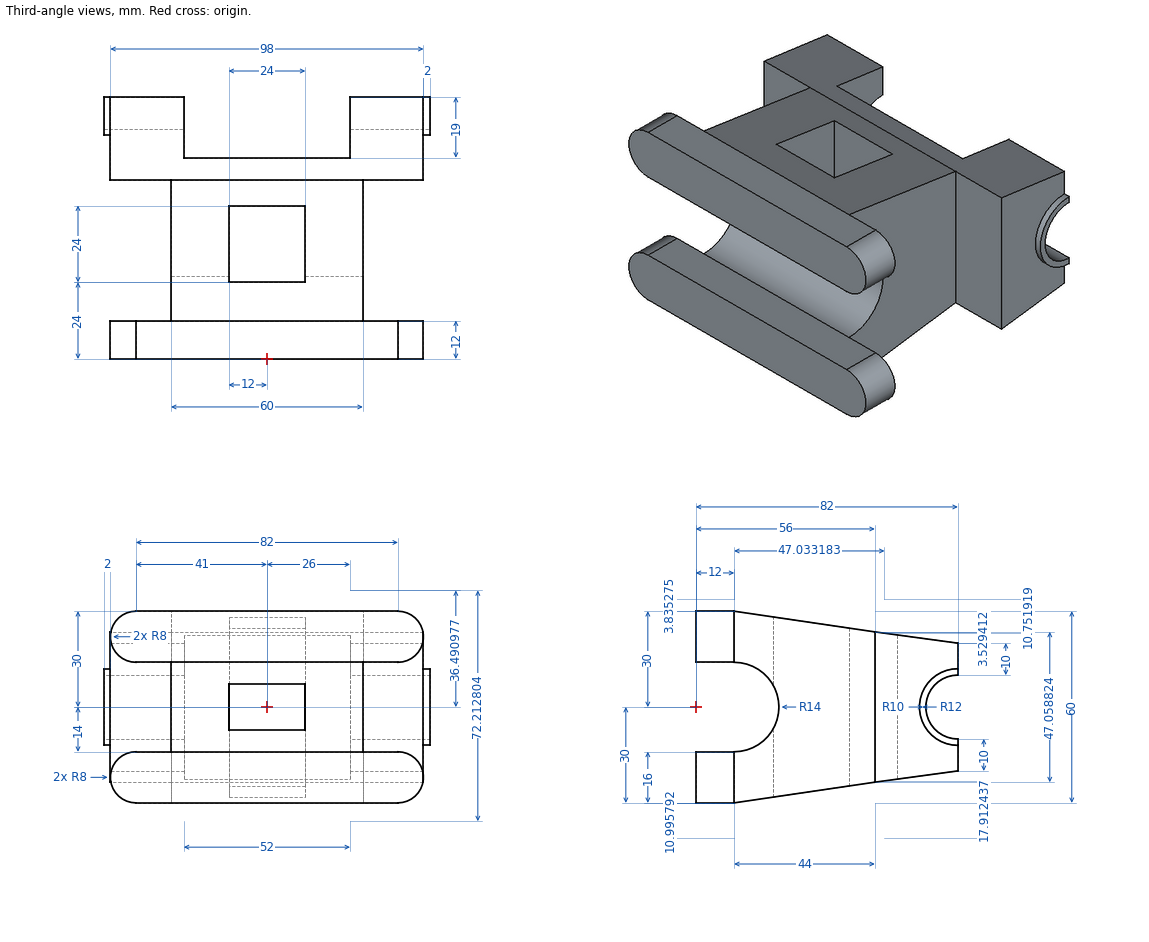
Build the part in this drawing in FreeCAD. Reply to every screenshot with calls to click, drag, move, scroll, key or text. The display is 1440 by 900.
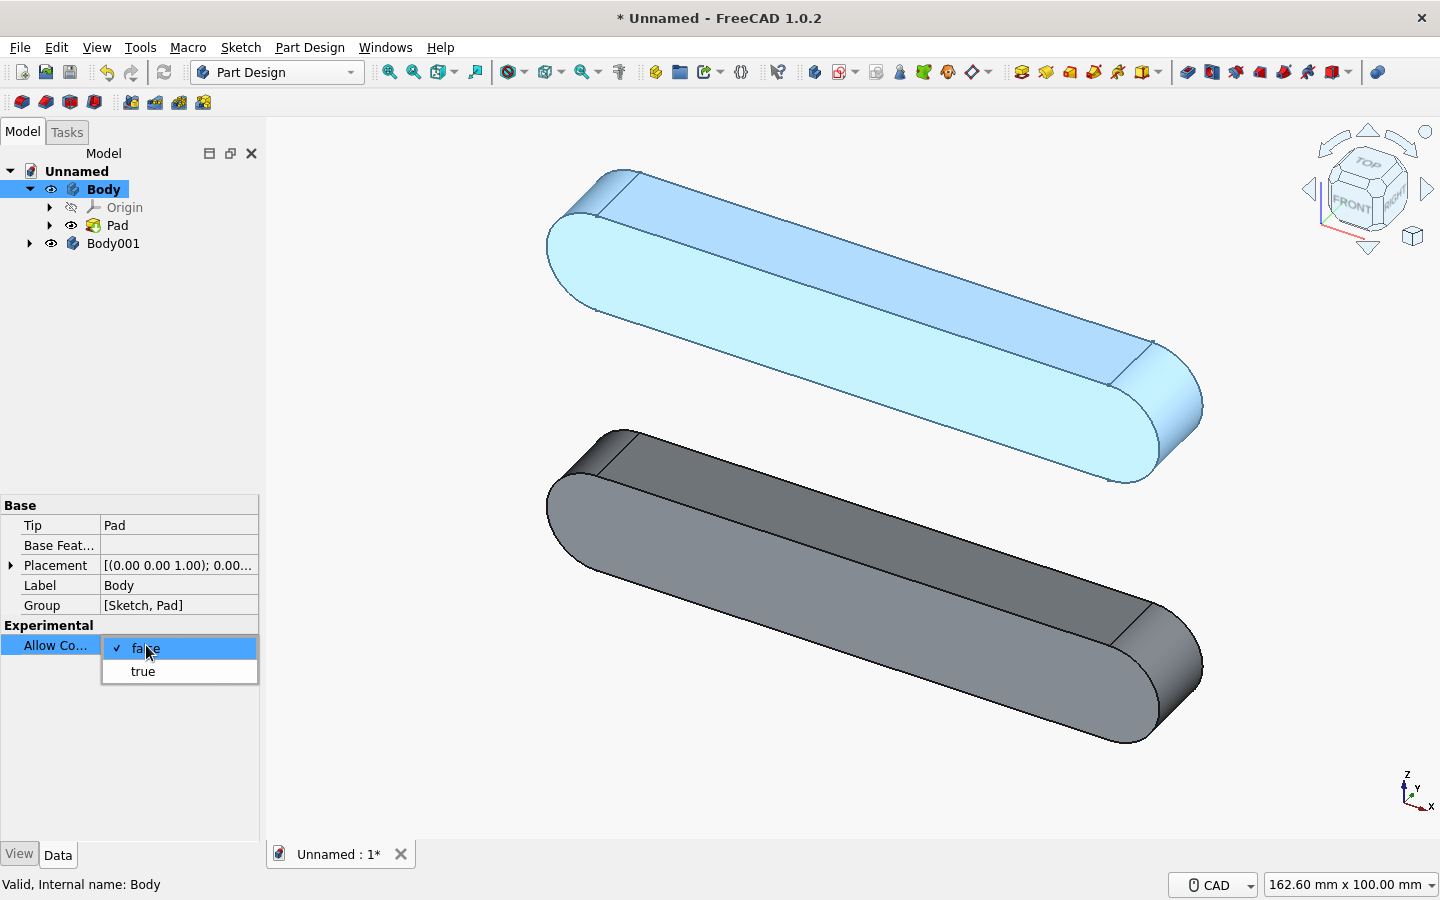
click(179, 672)
key(Return)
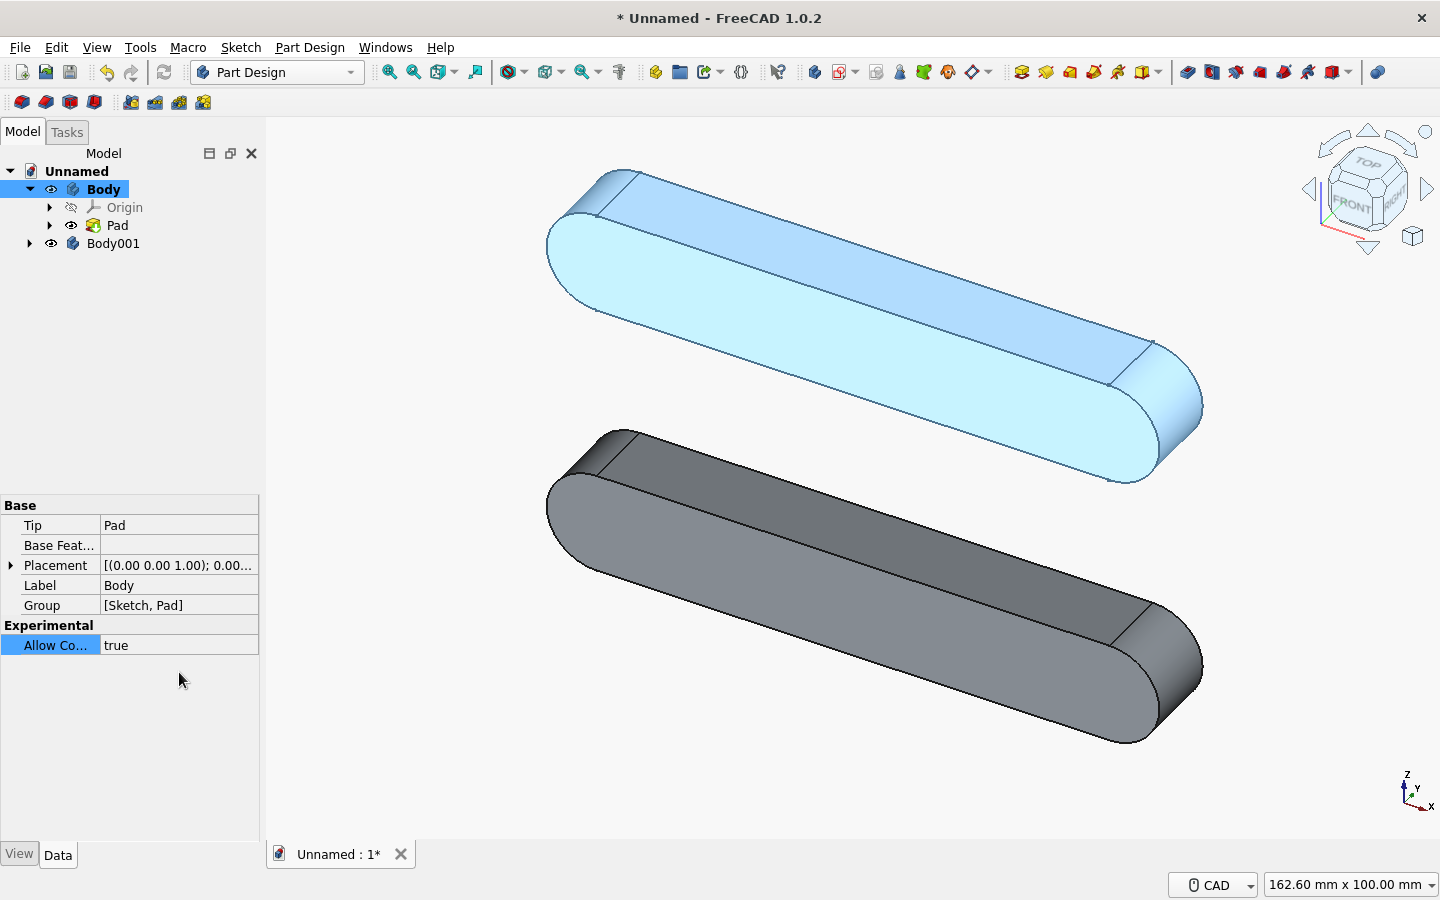
click(96, 243)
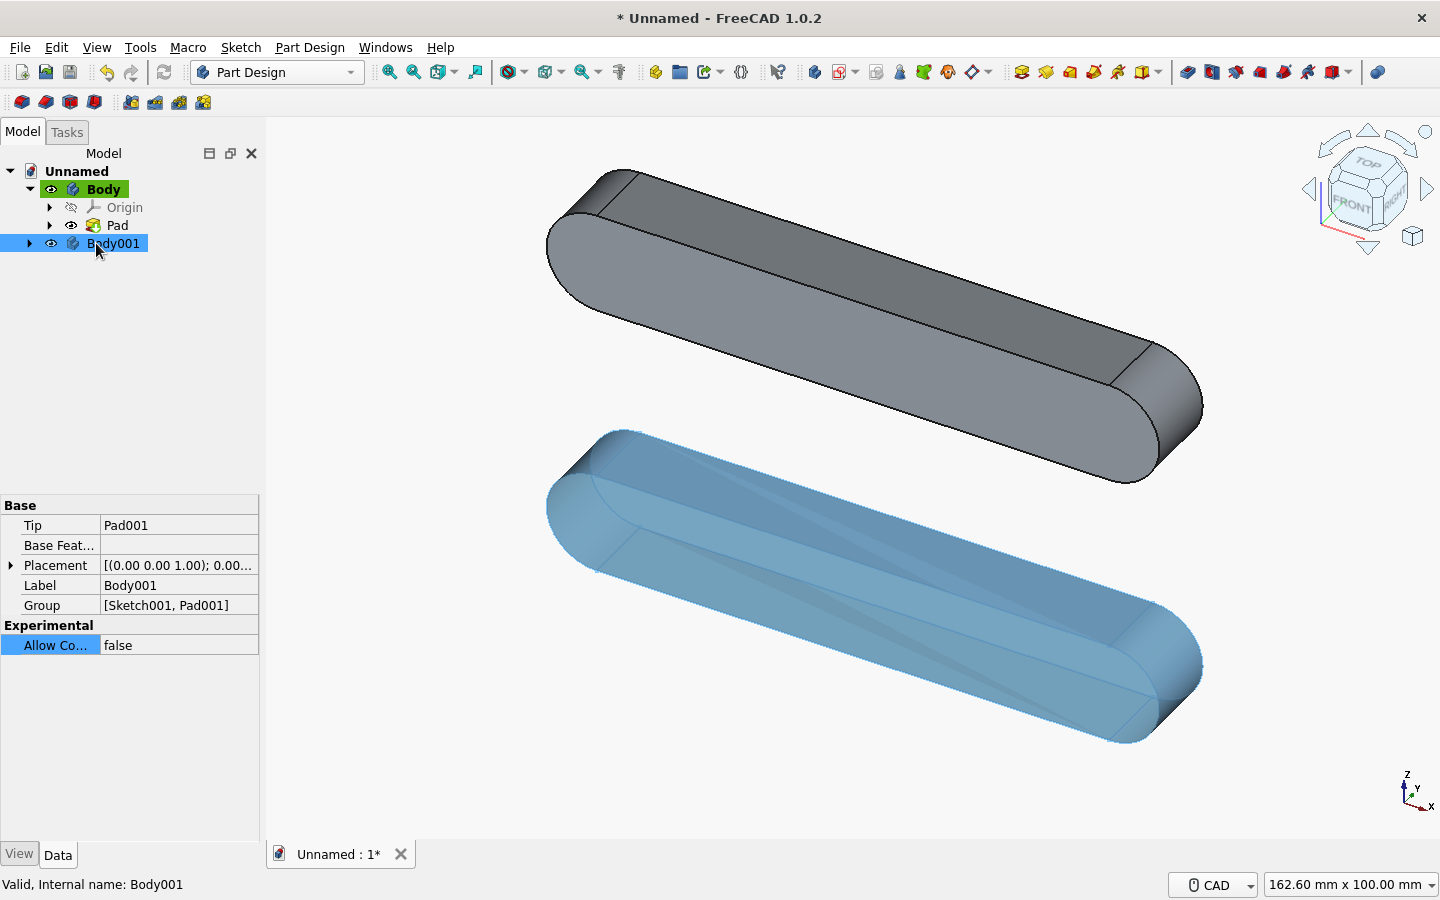
click(1378, 72)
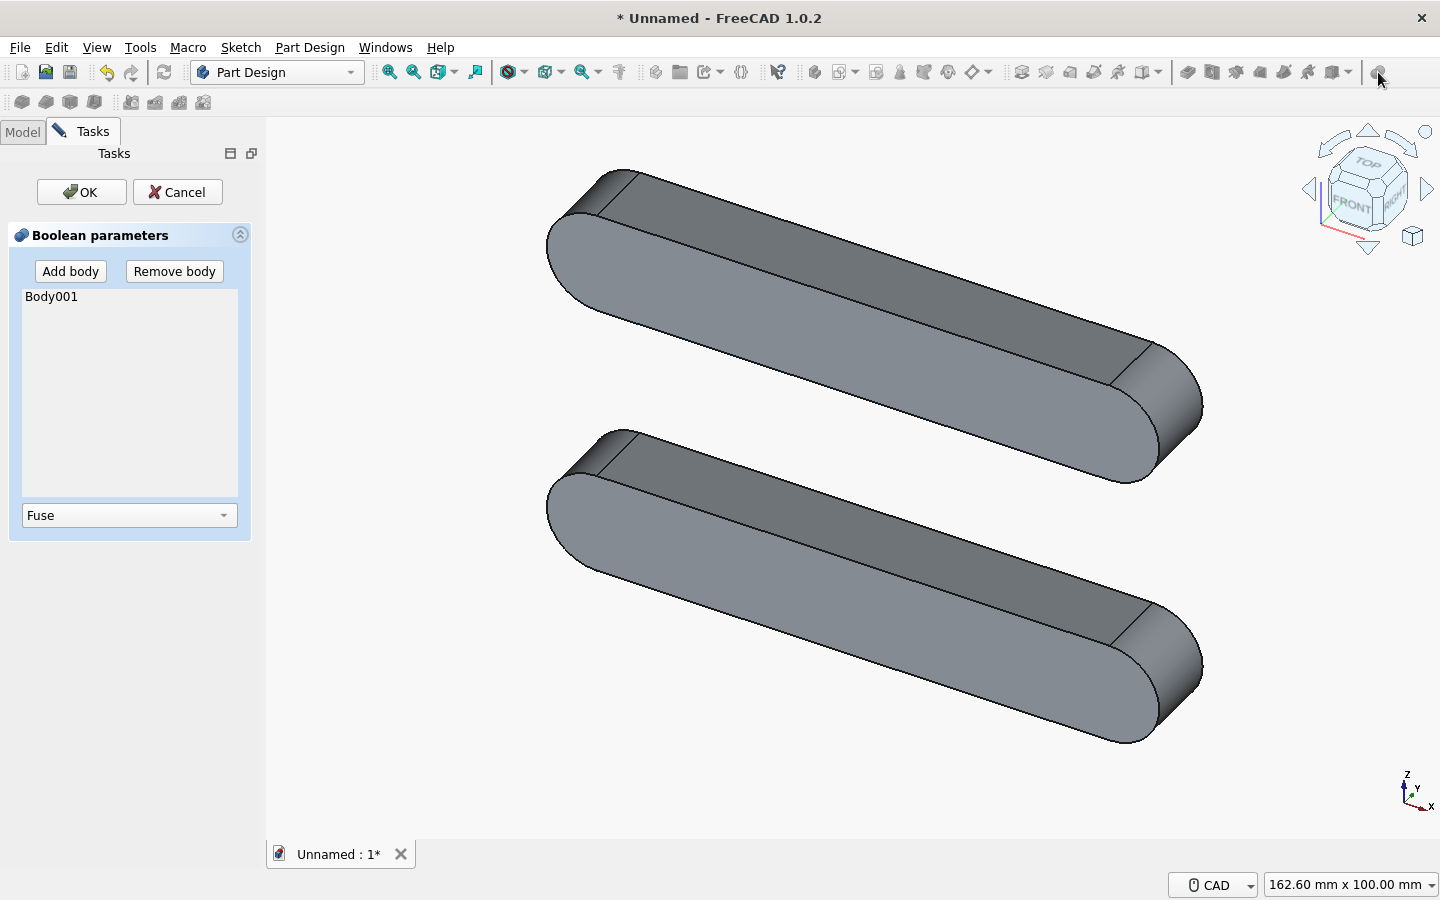
click(82, 192)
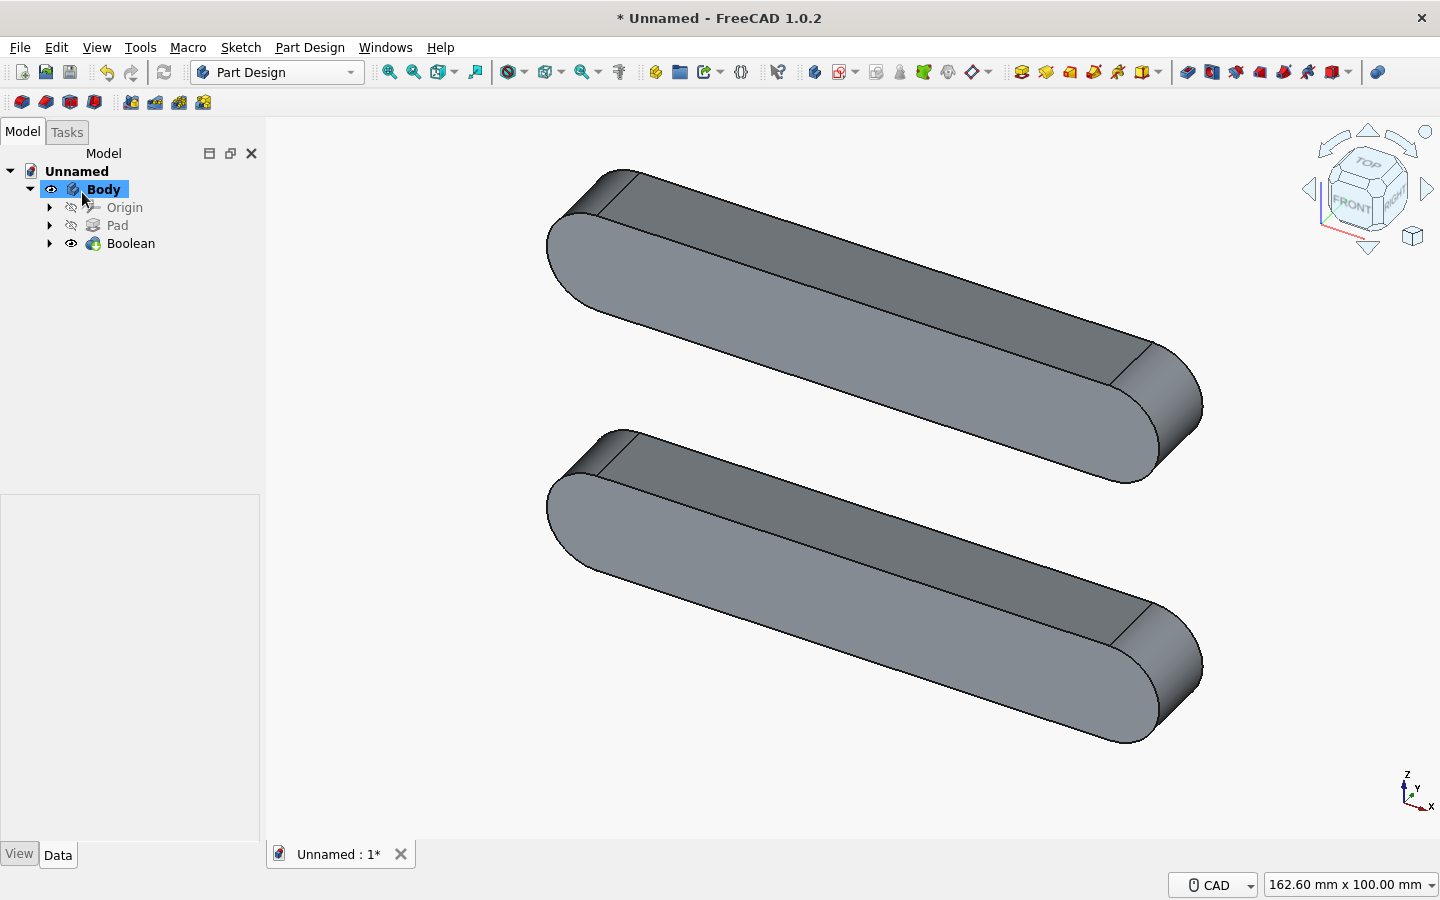
click(50, 207)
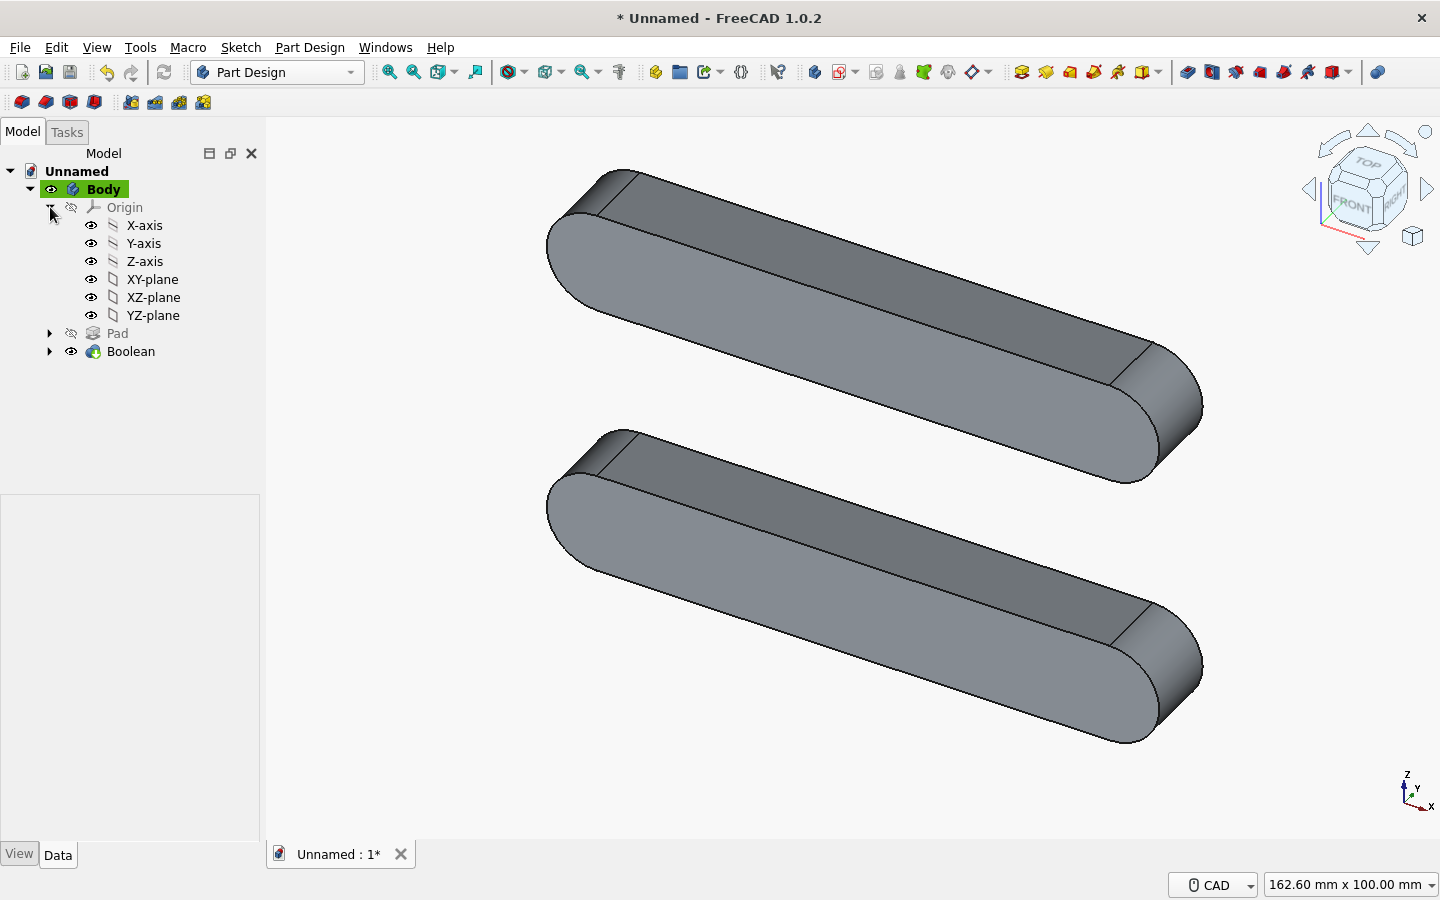
click(136, 315)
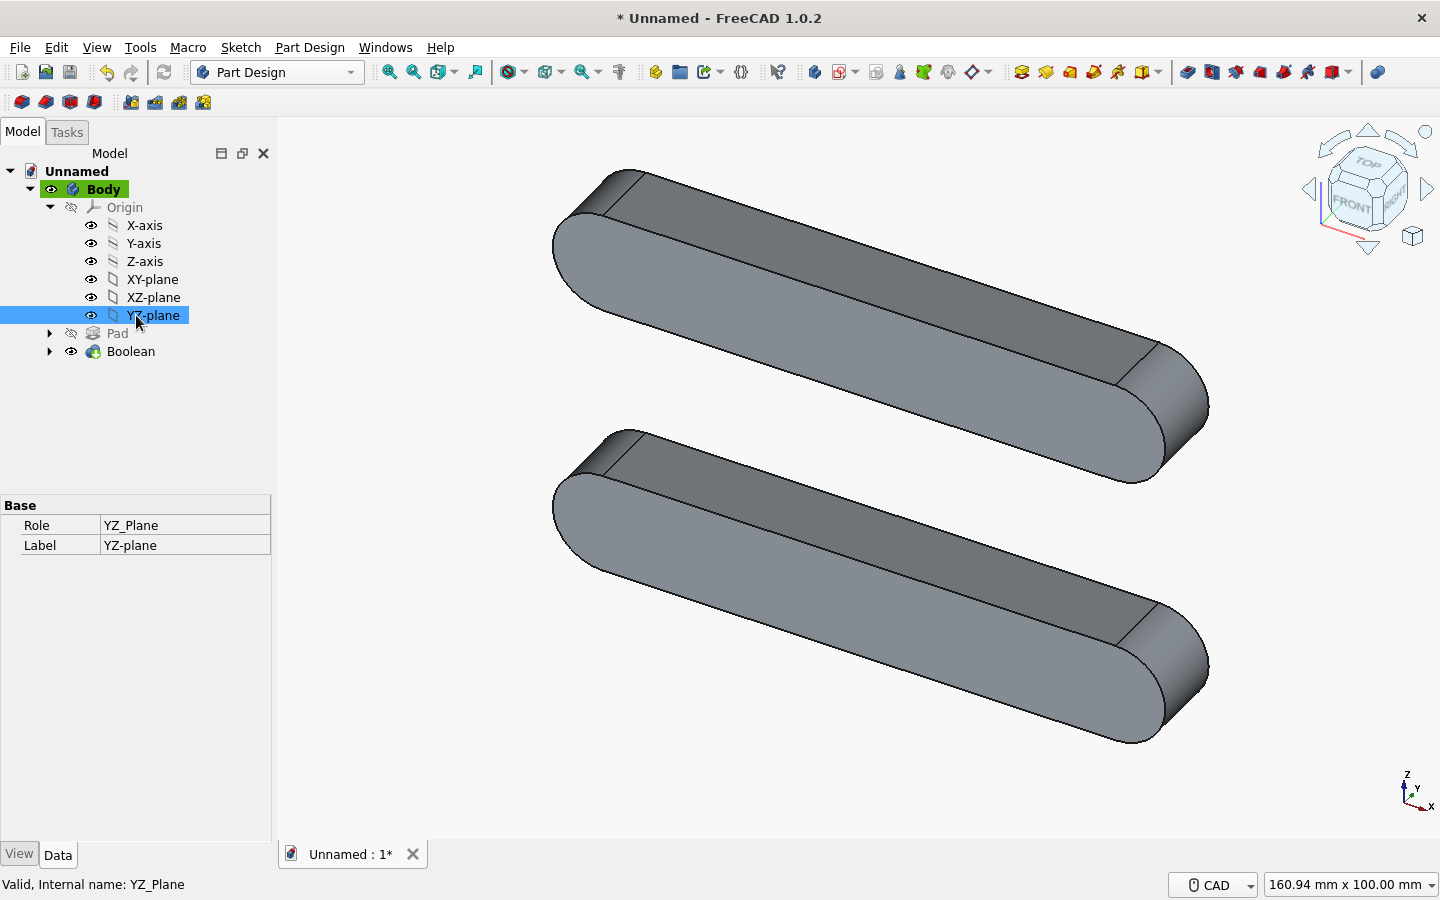
click(972, 72)